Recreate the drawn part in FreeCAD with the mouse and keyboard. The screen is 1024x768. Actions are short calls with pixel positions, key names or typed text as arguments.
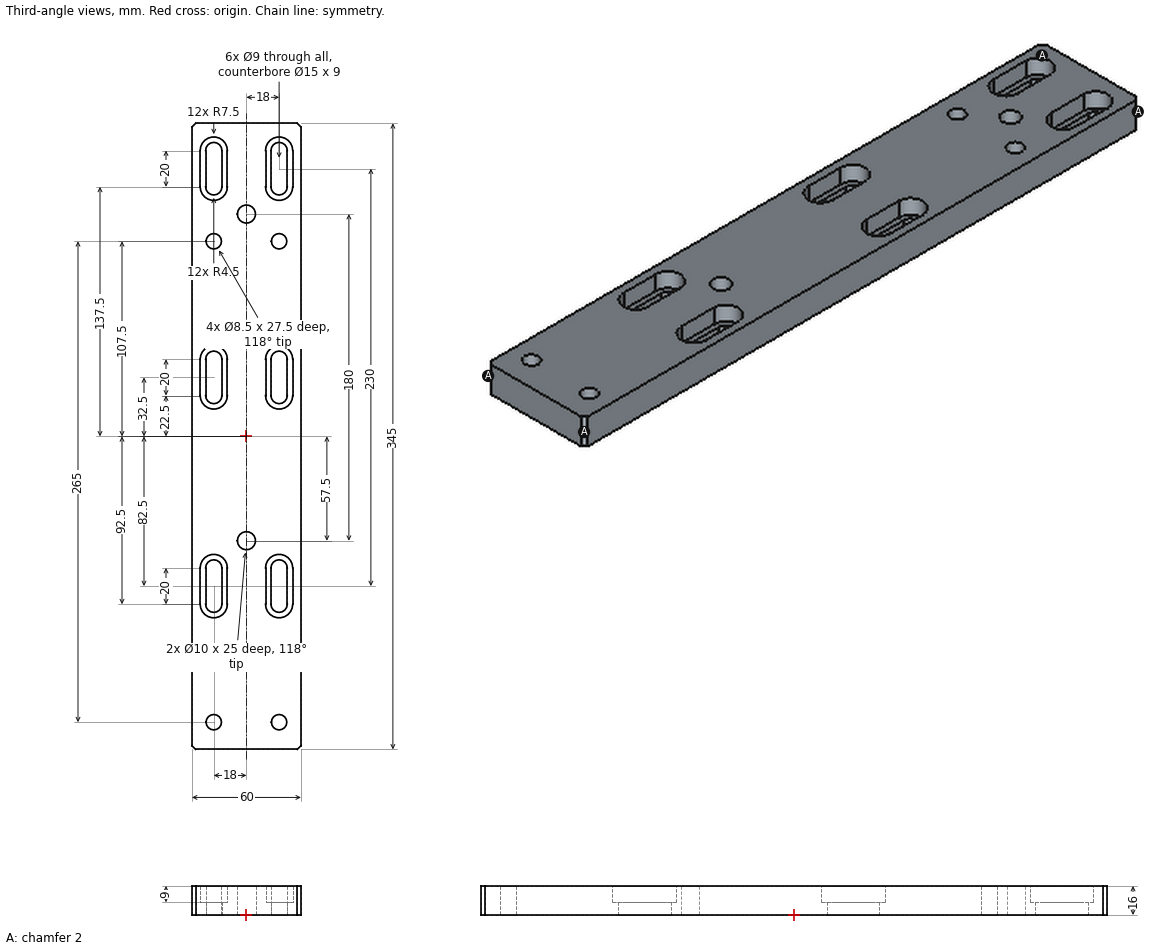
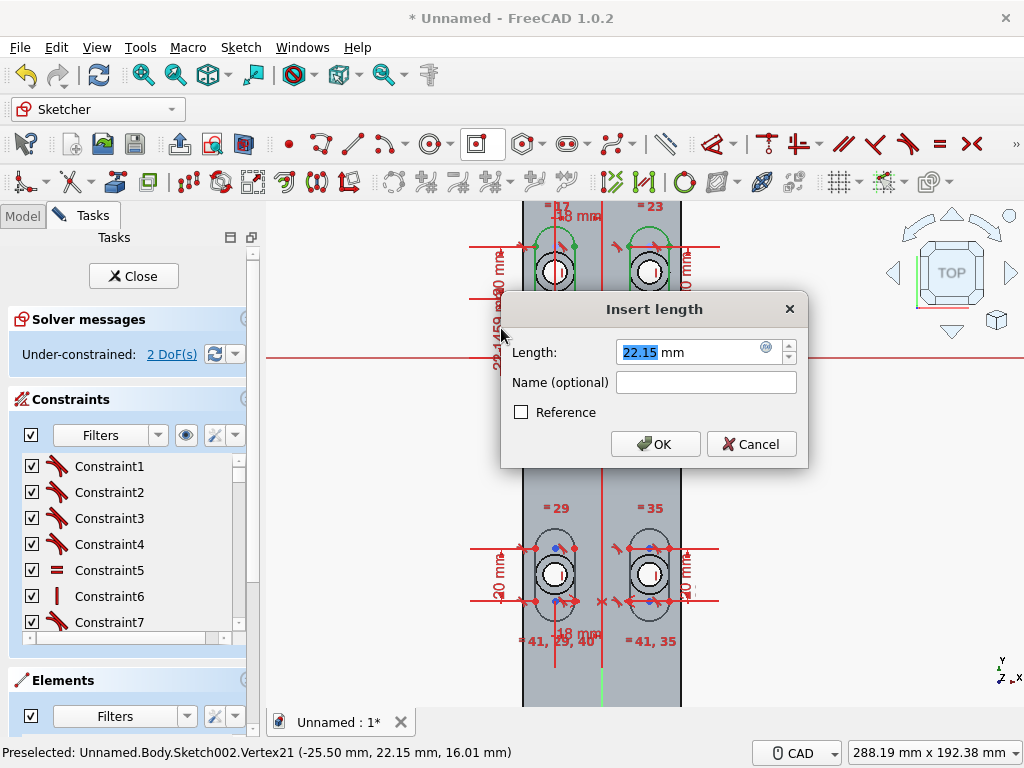
text(22.5)
key(Return)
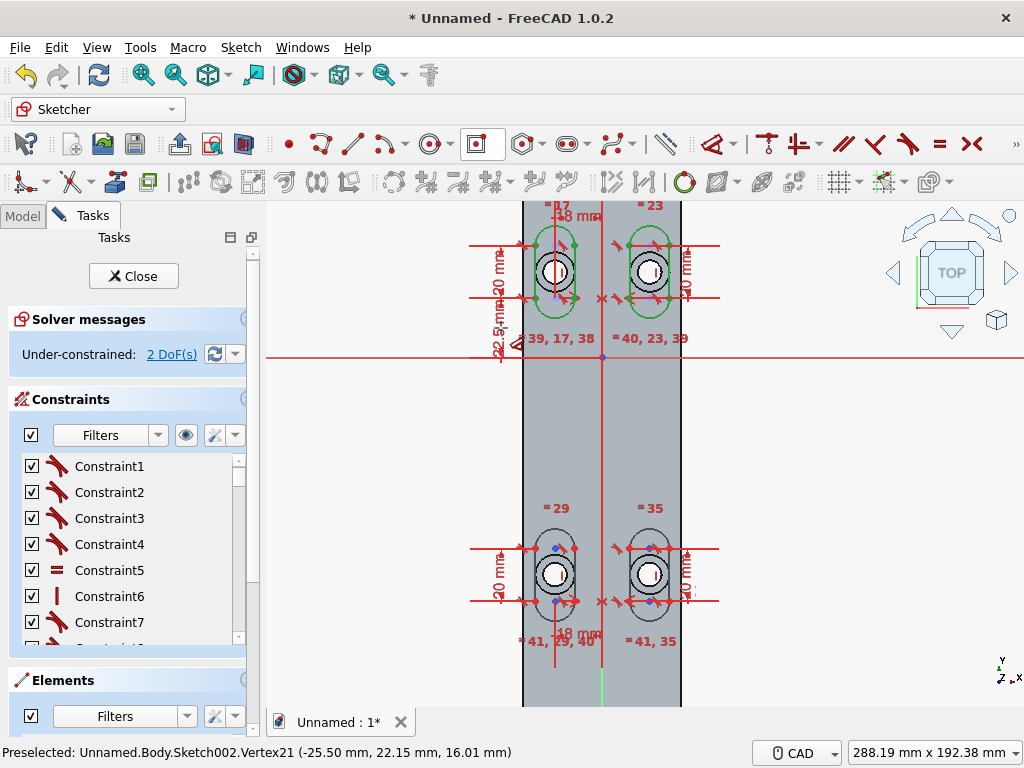
click(535, 601)
click(501, 479)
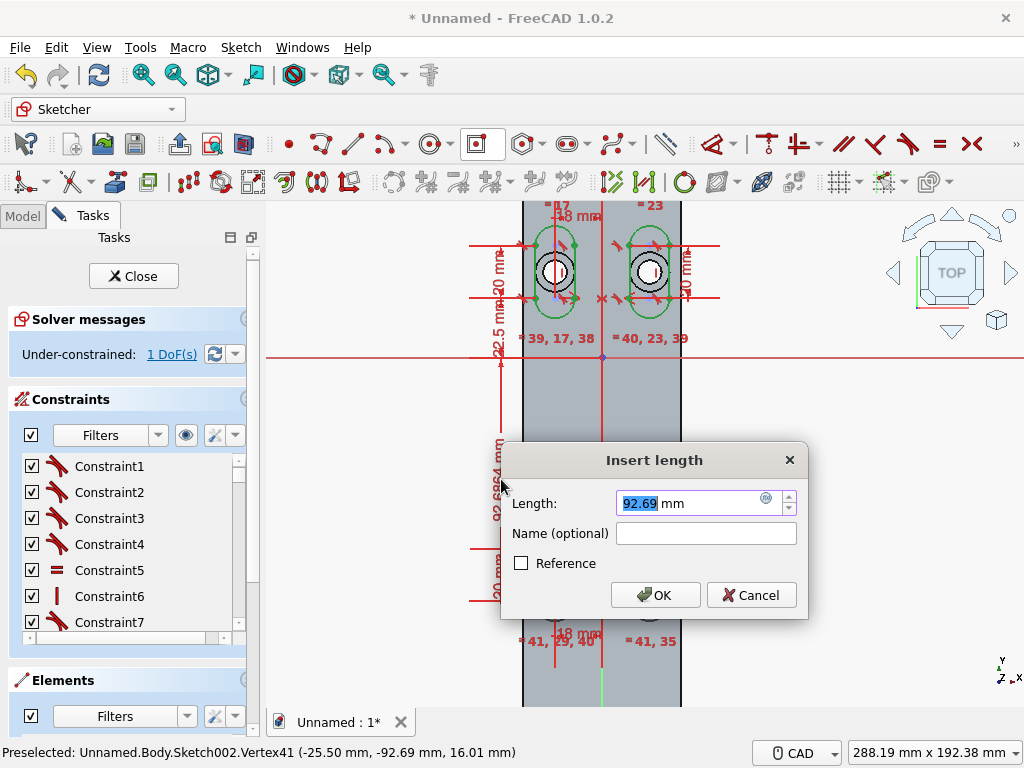
text(92.5)
key(Return)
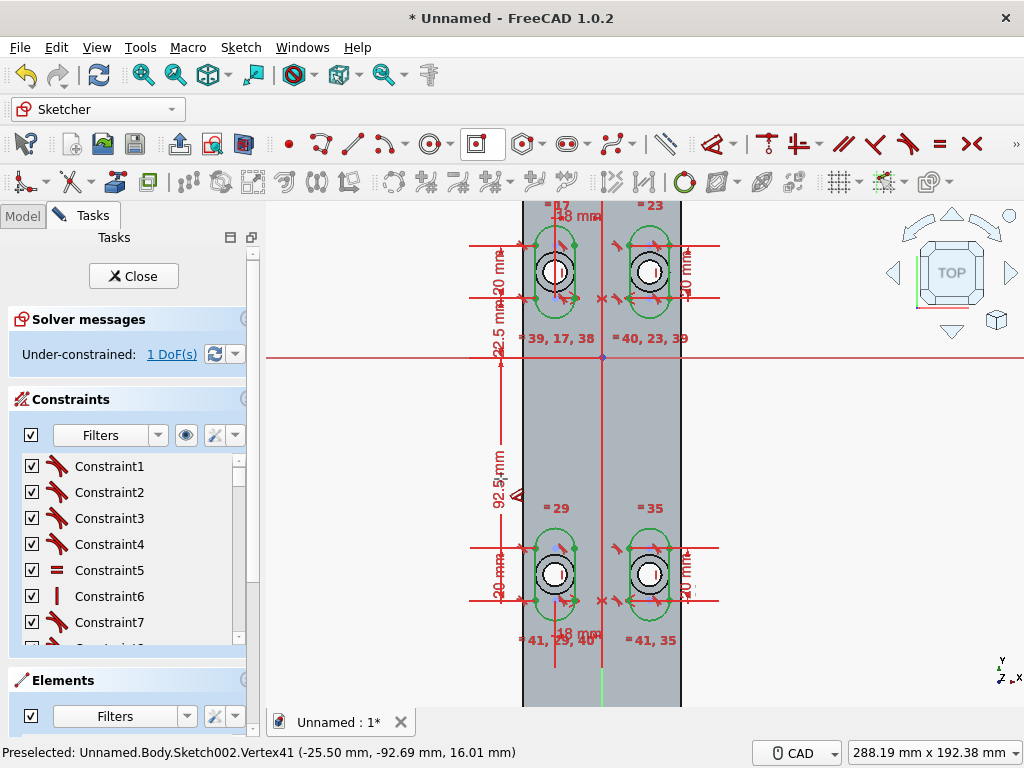
scroll(555, 602, down, 4)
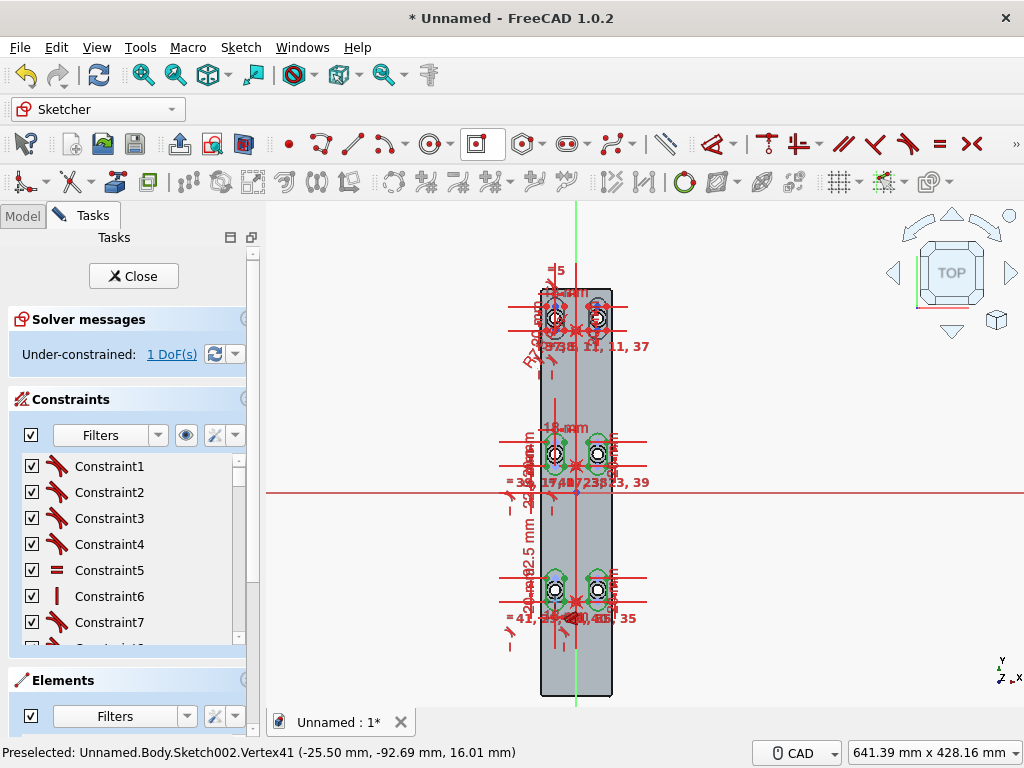
scroll(546, 331, up, 2)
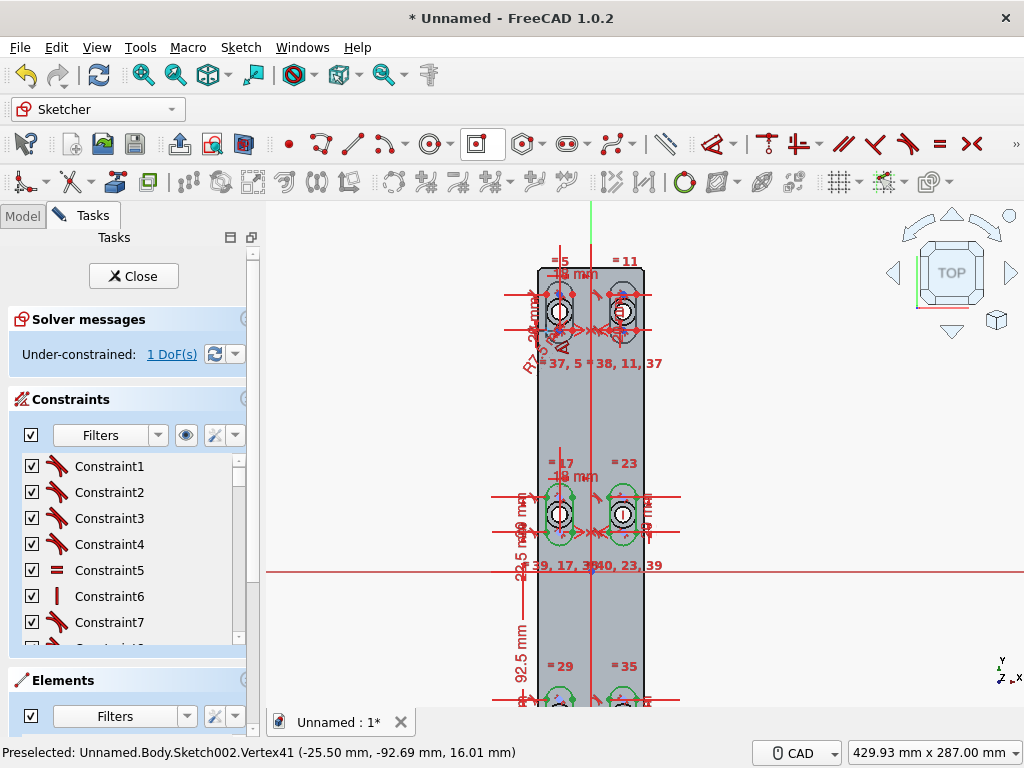
click(546, 330)
click(512, 451)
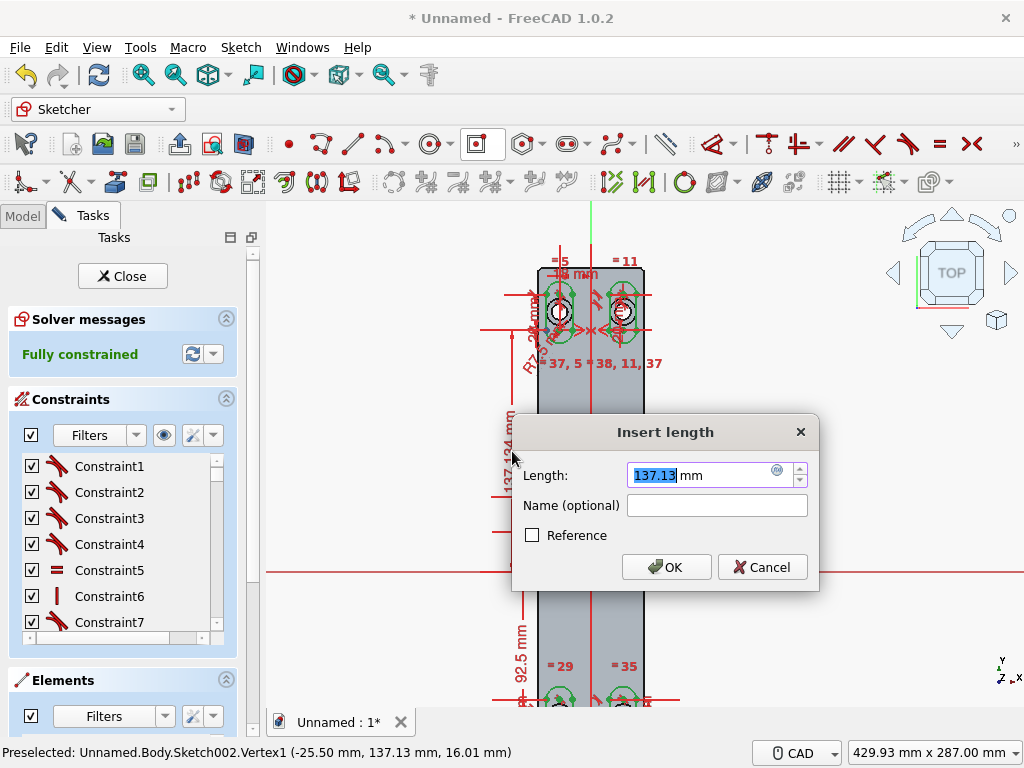
text(137.5)
key(Return)
key(Escape)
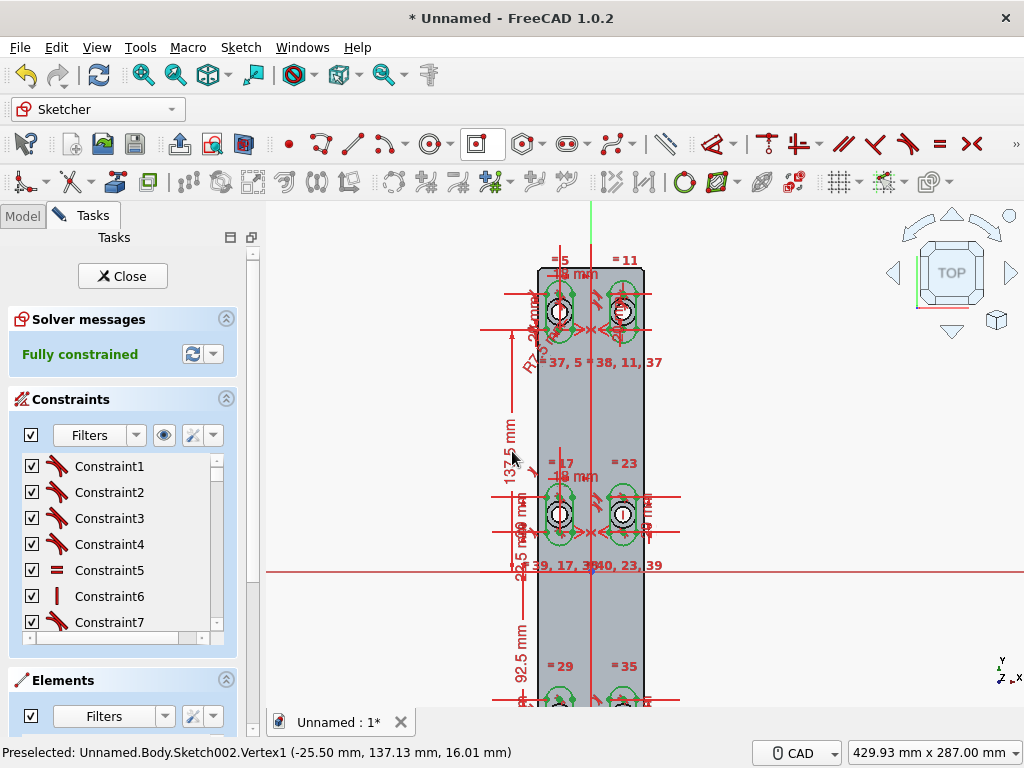
click(123, 276)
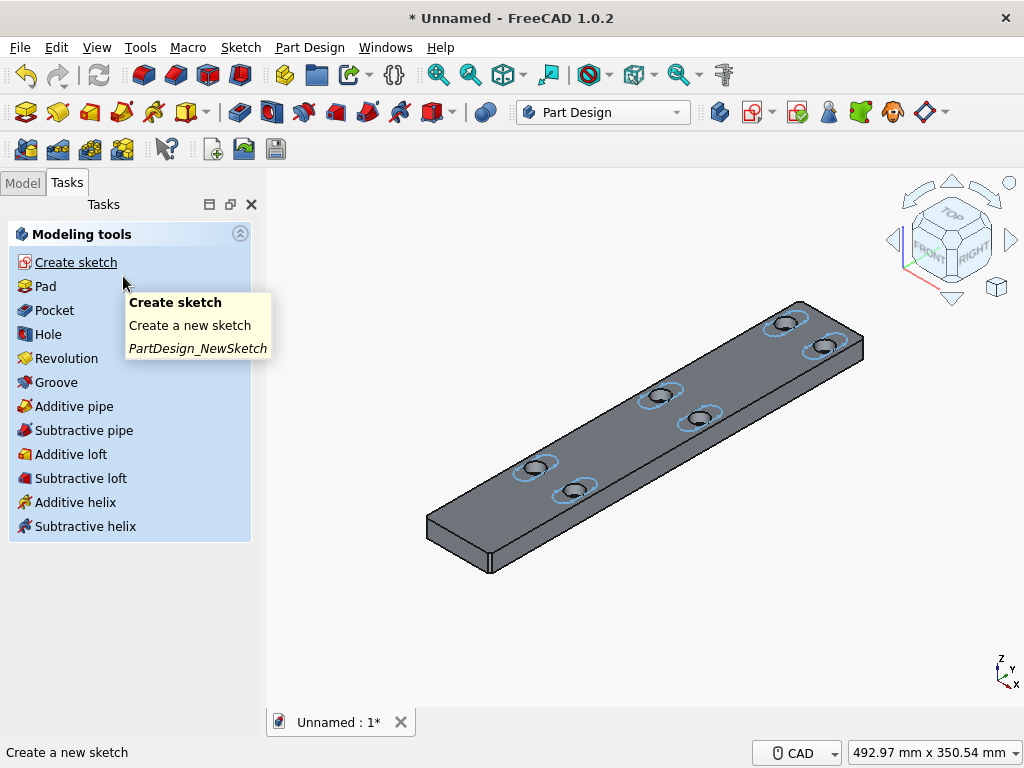
click(240, 112)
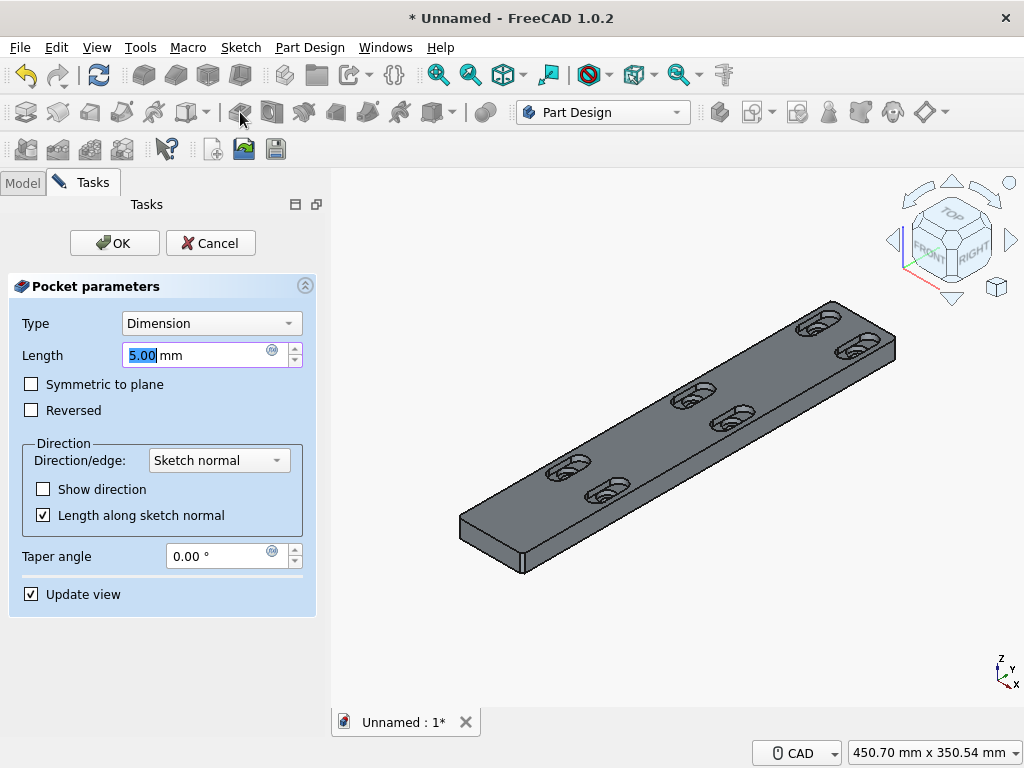
text(9)
key(Tab)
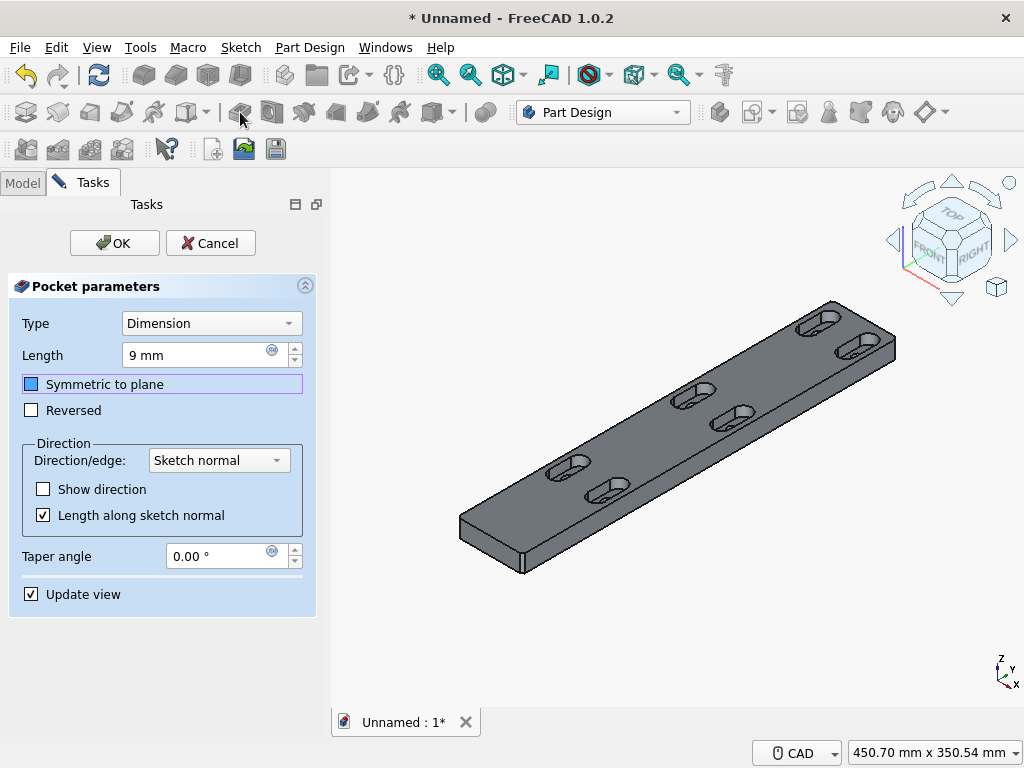
click(115, 243)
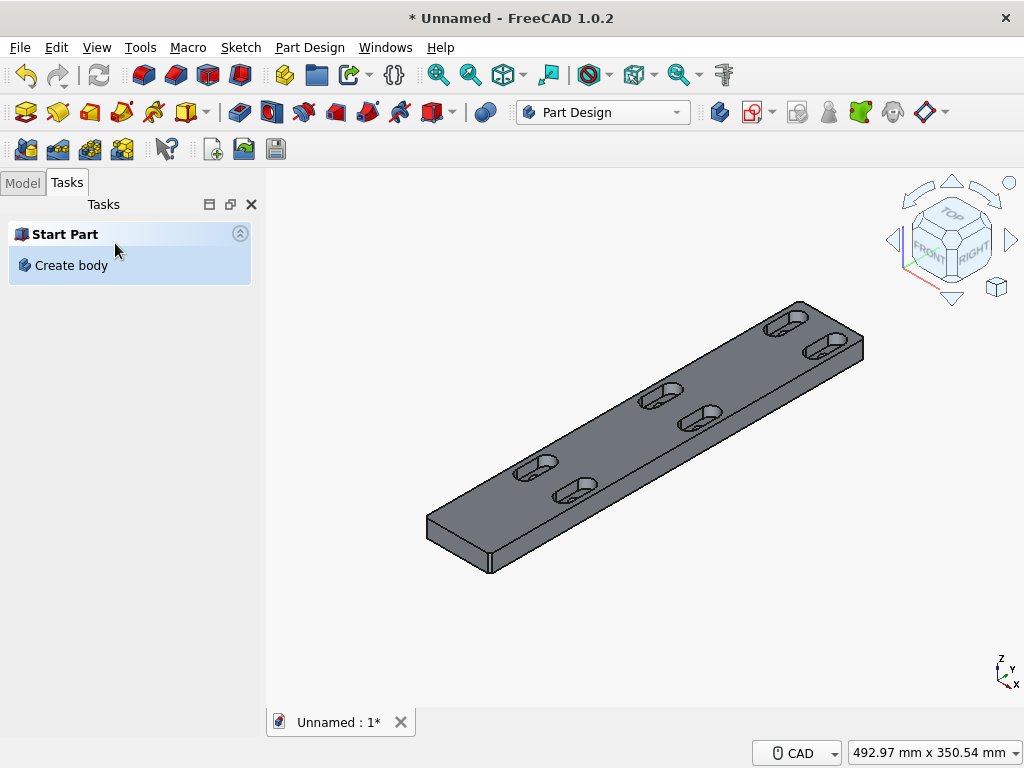
key(2)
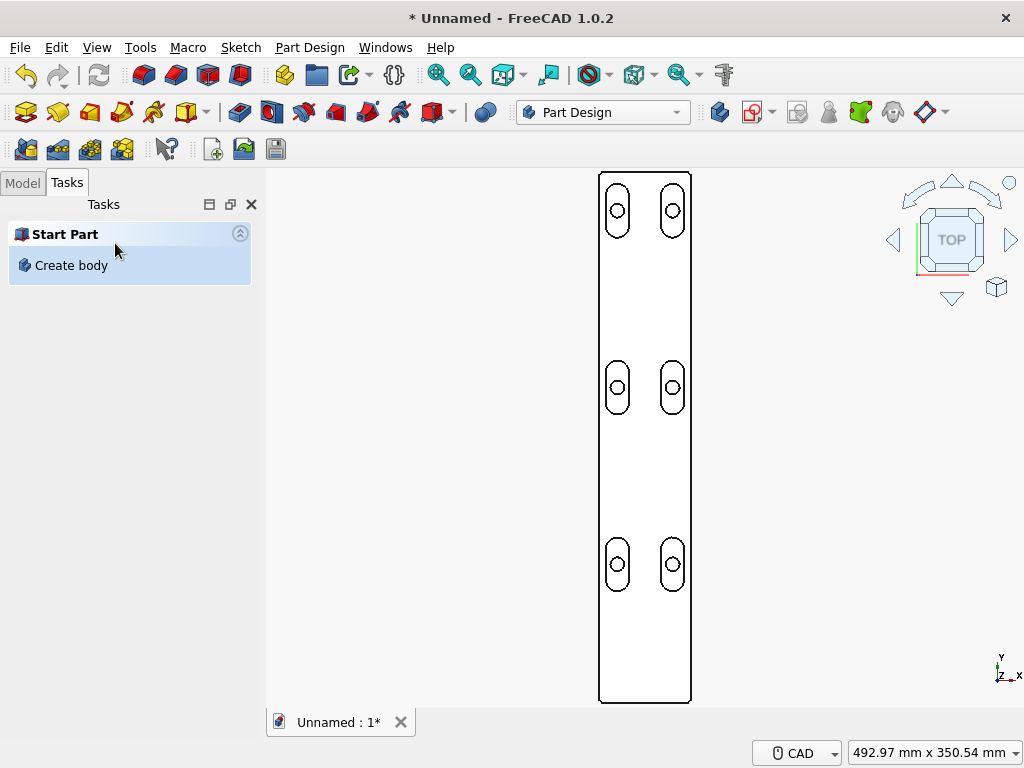
click(673, 225)